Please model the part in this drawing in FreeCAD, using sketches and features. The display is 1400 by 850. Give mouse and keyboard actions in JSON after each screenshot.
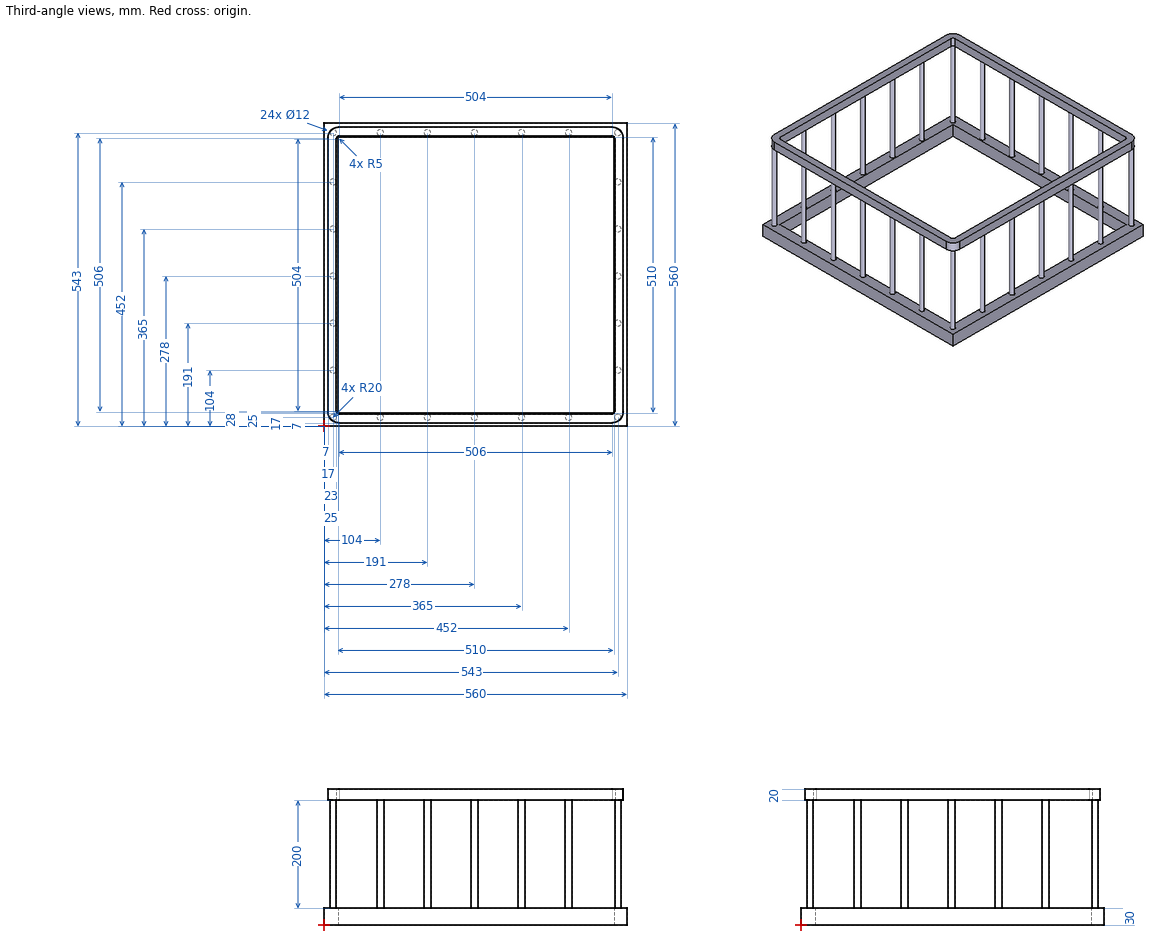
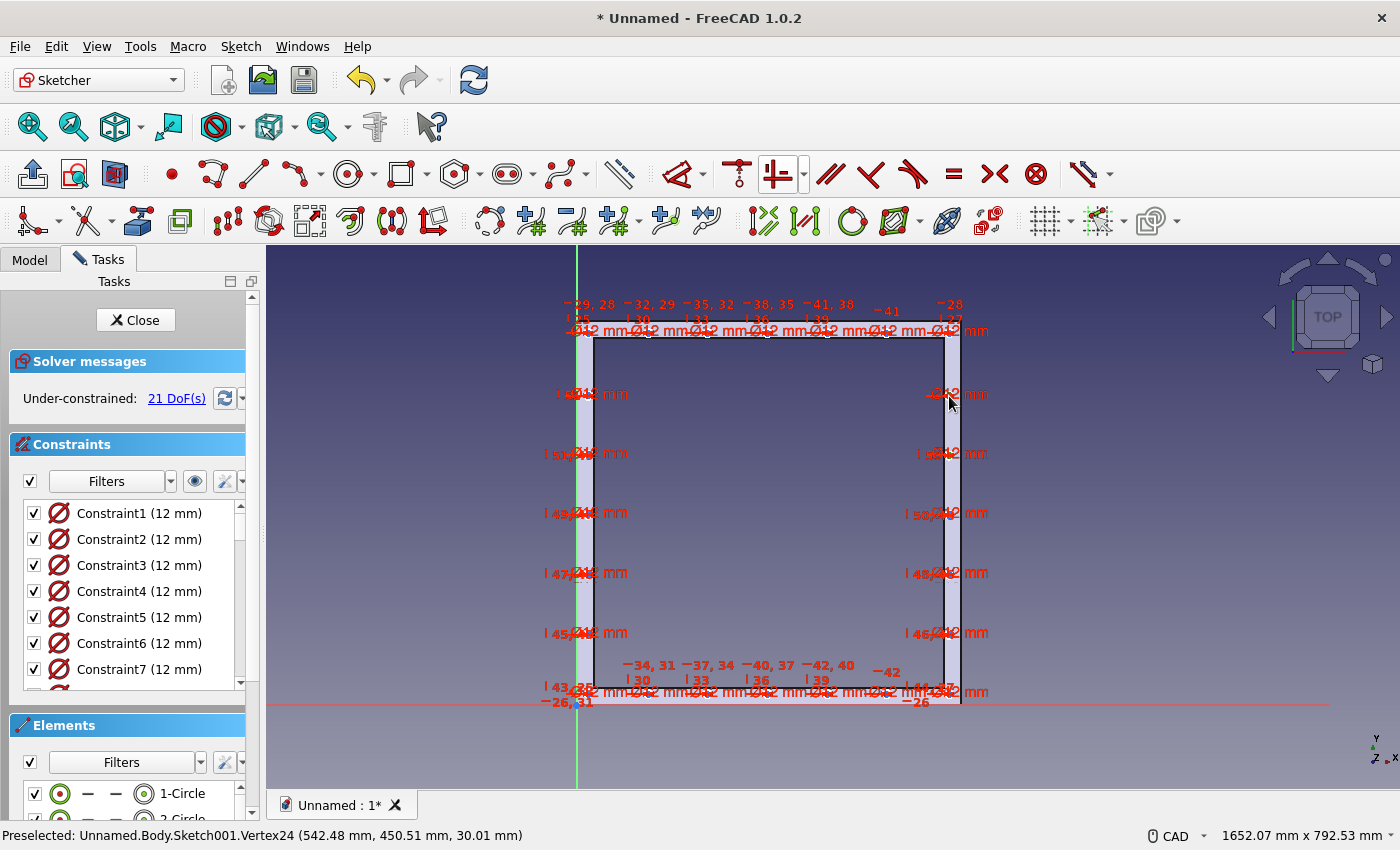
{"action": "key", "text": "v"}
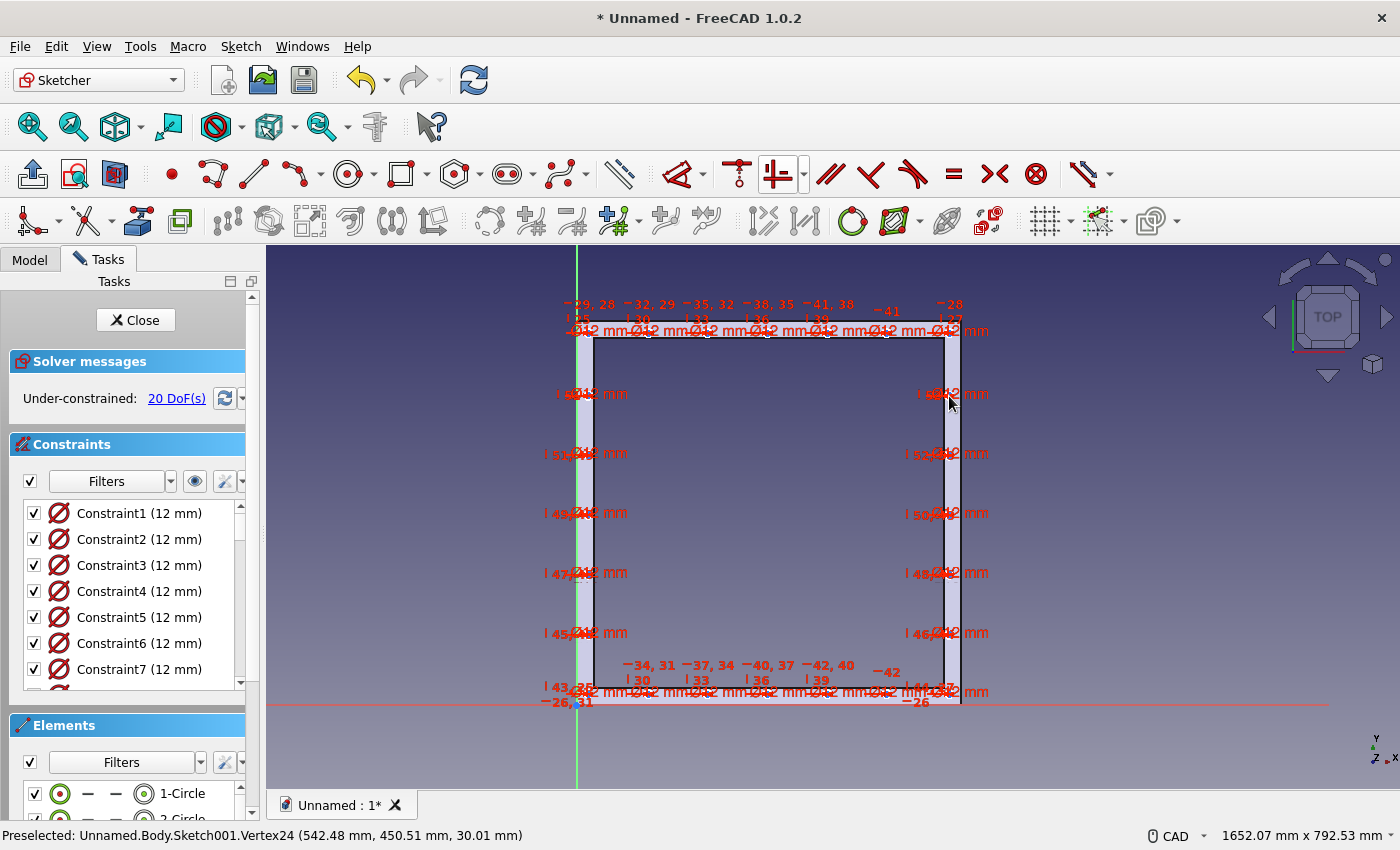
{"action": "left_click", "coordinate": [676, 174]}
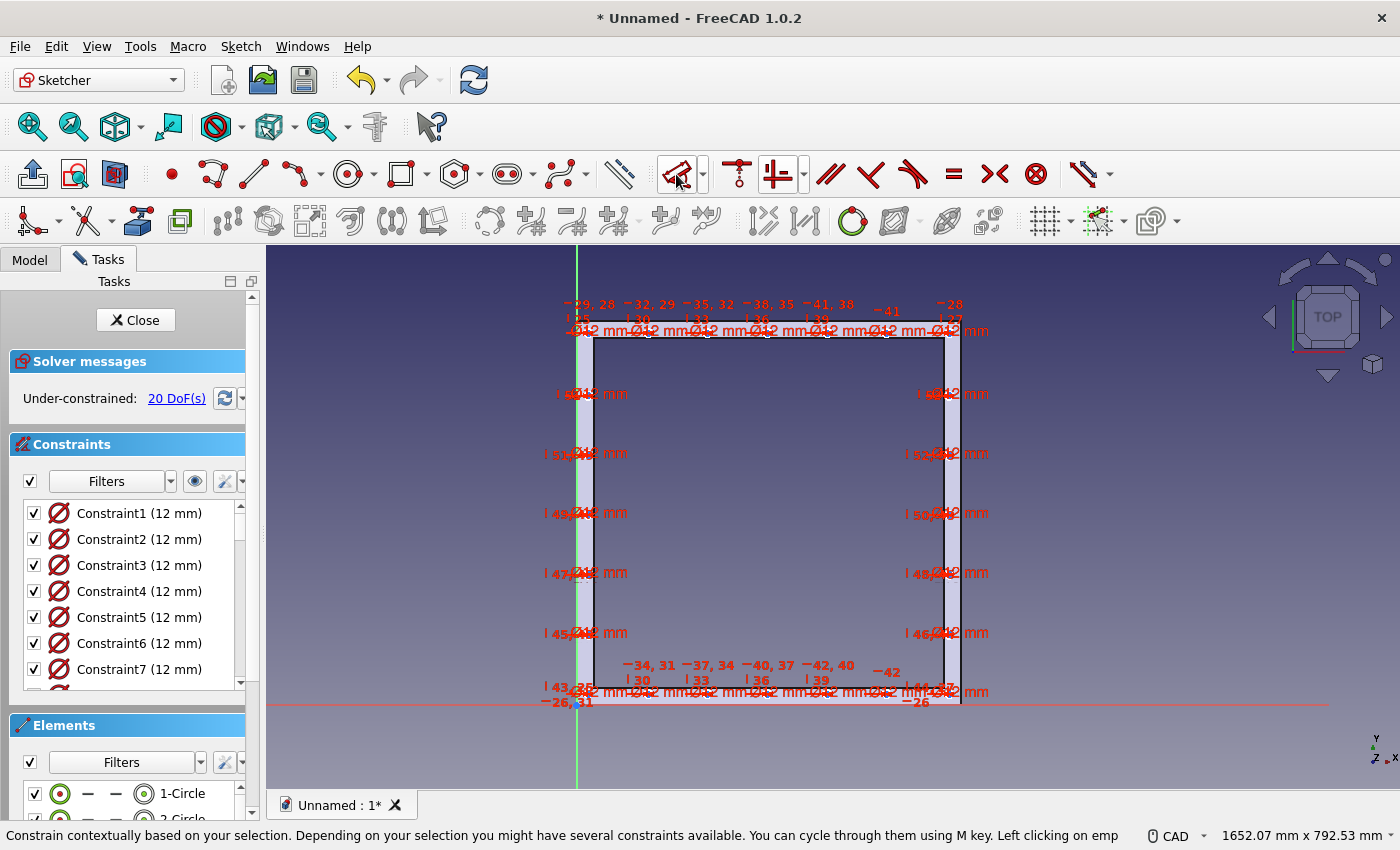
{"action": "scroll", "coordinate": [588, 333], "scroll_direction": "up", "scroll_amount": 7}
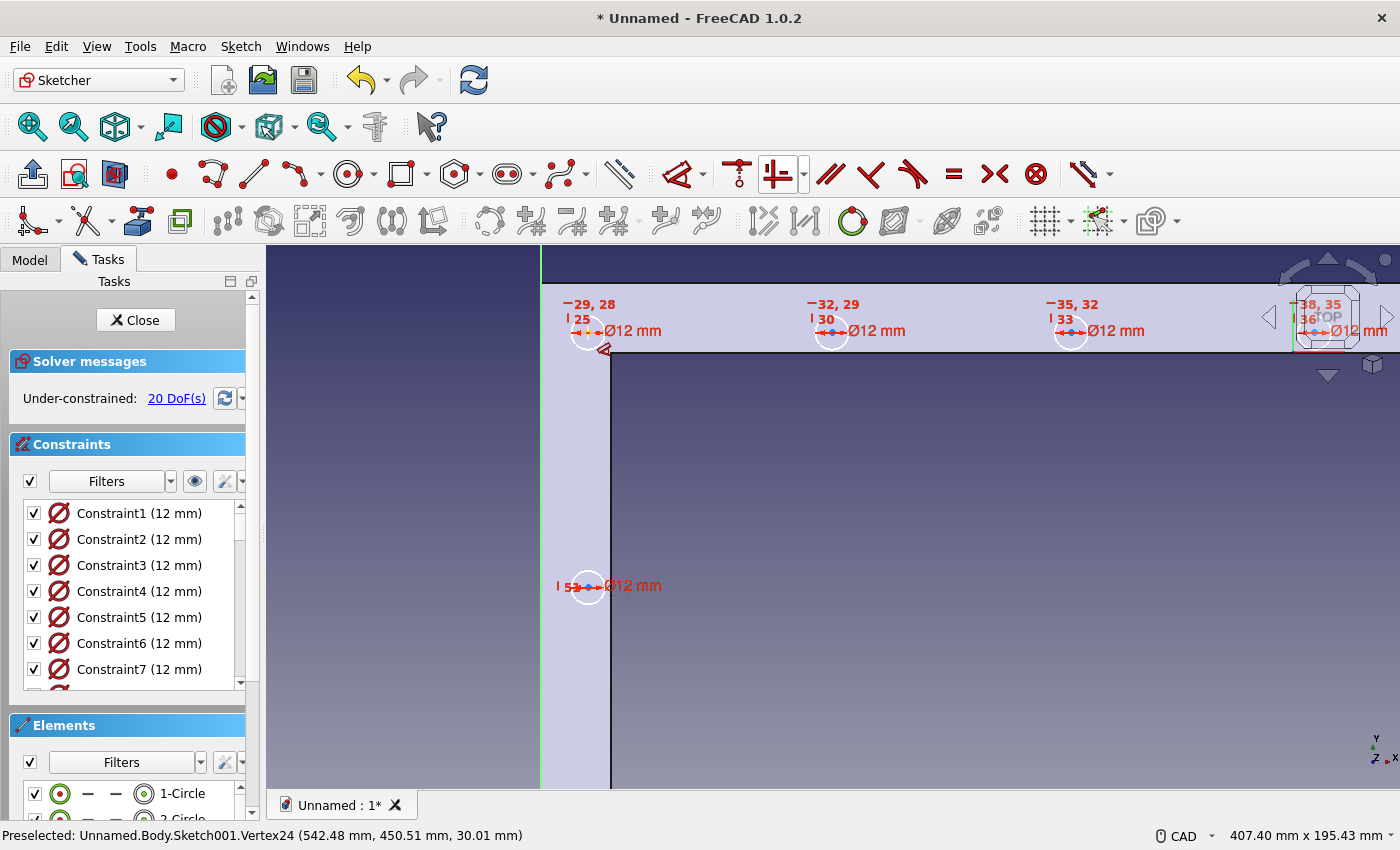
{"action": "left_click", "coordinate": [588, 333]}
{"action": "left_click", "coordinate": [565, 299]}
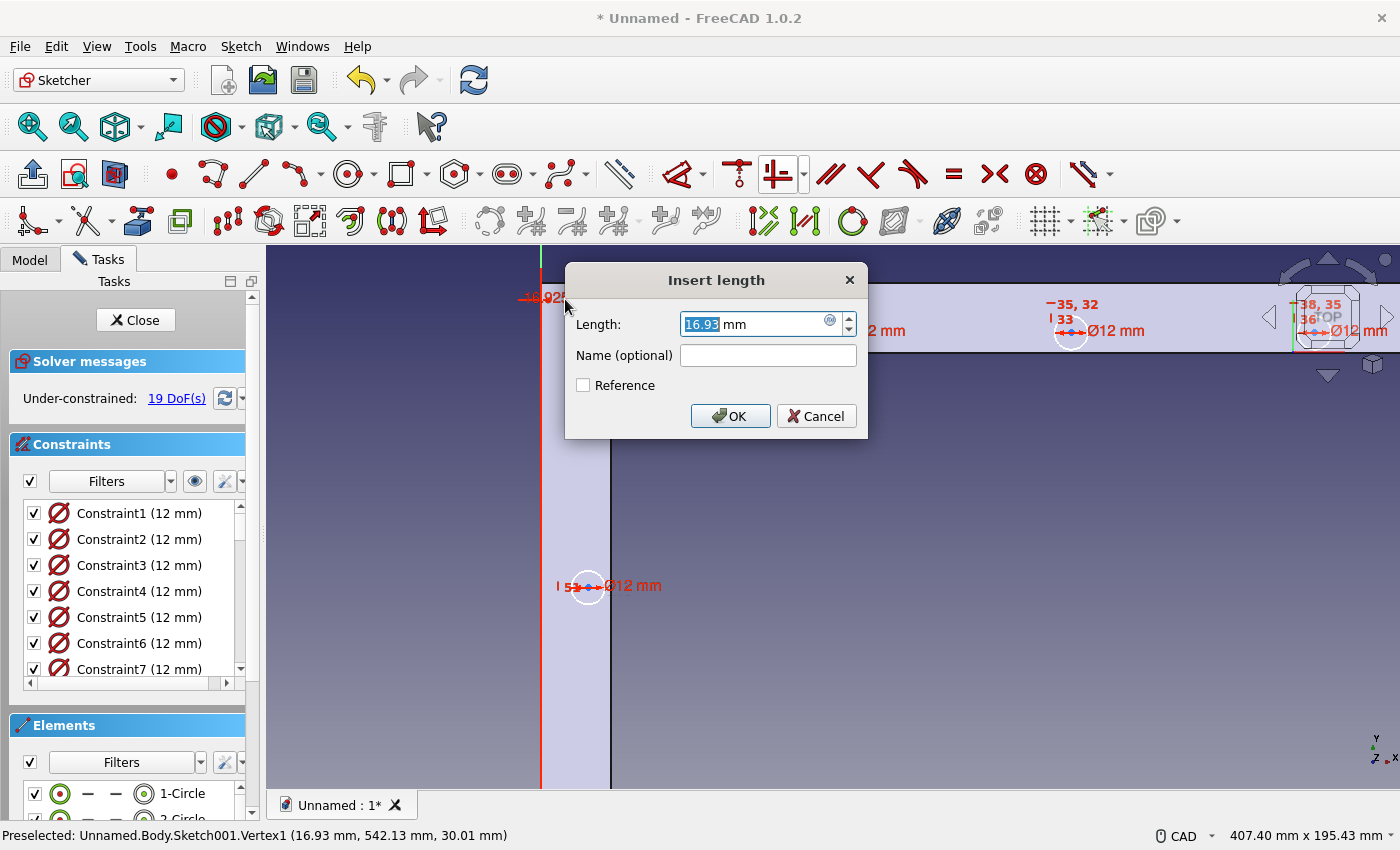
{"action": "type", "text": "17"}
{"action": "key", "text": "Return"}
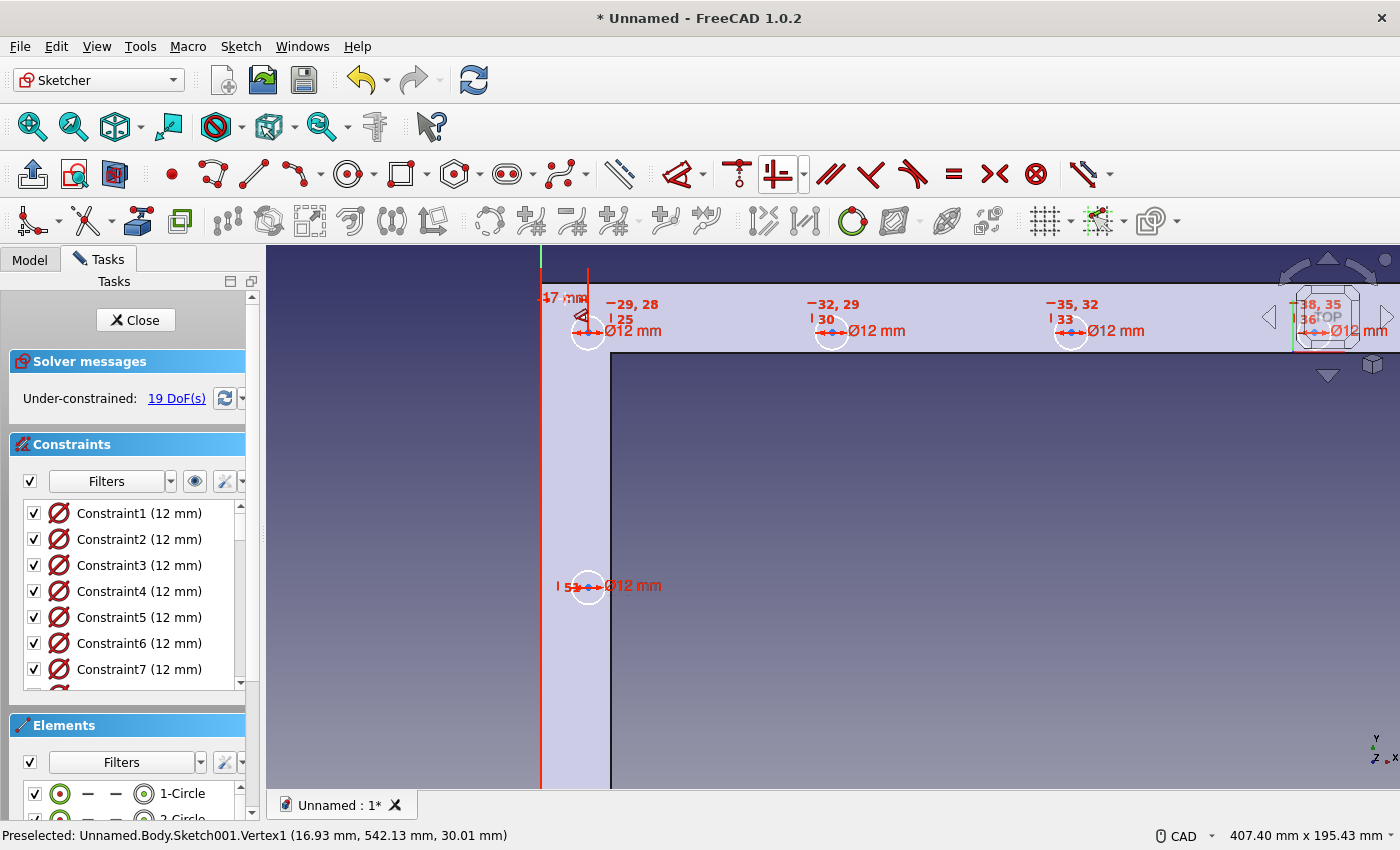
{"action": "scroll", "coordinate": [588, 333], "scroll_direction": "down", "scroll_amount": 7}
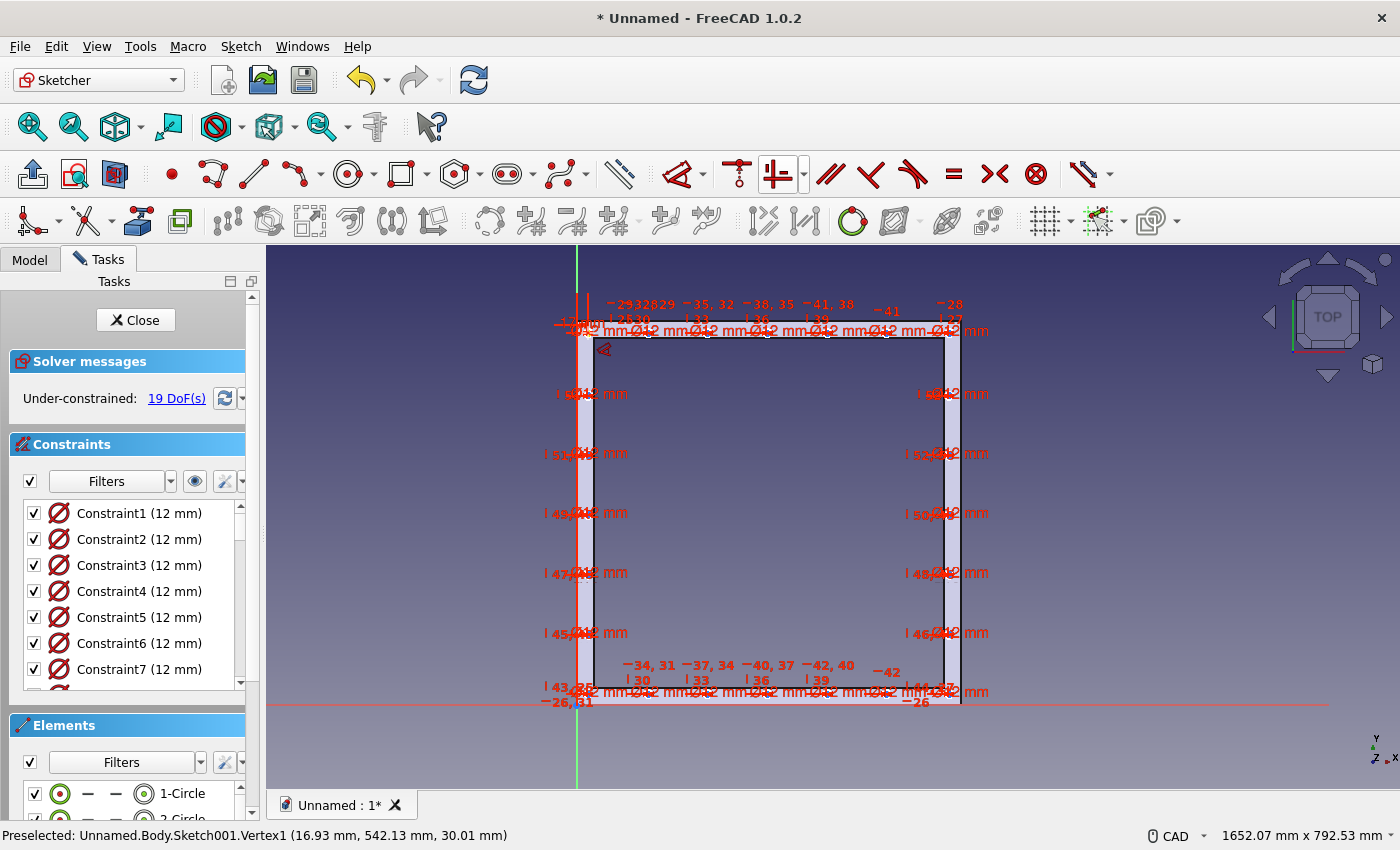
{"action": "scroll", "coordinate": [588, 694], "scroll_direction": "up", "scroll_amount": 7}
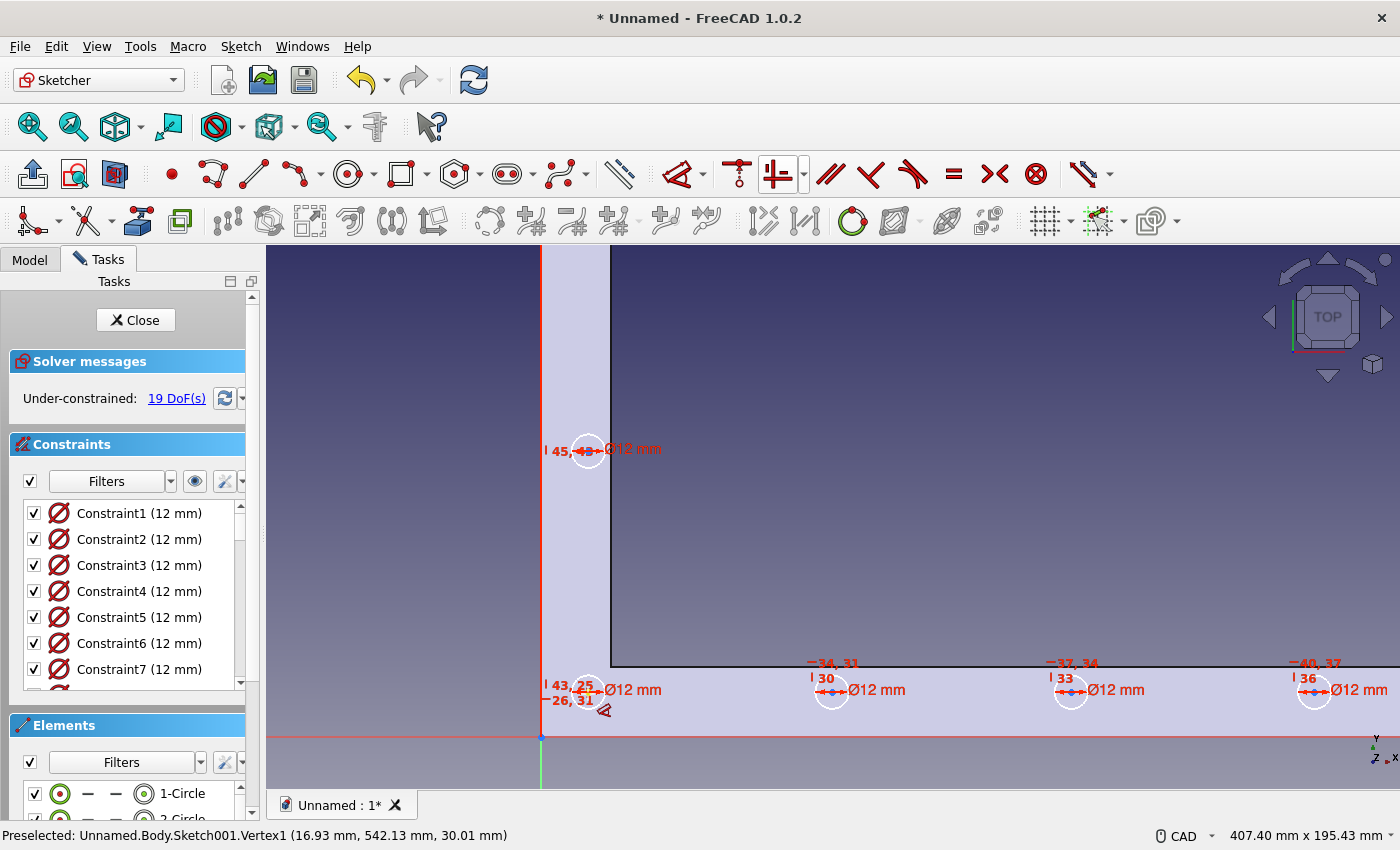
{"action": "left_click", "coordinate": [588, 692]}
{"action": "left_click", "coordinate": [507, 715]}